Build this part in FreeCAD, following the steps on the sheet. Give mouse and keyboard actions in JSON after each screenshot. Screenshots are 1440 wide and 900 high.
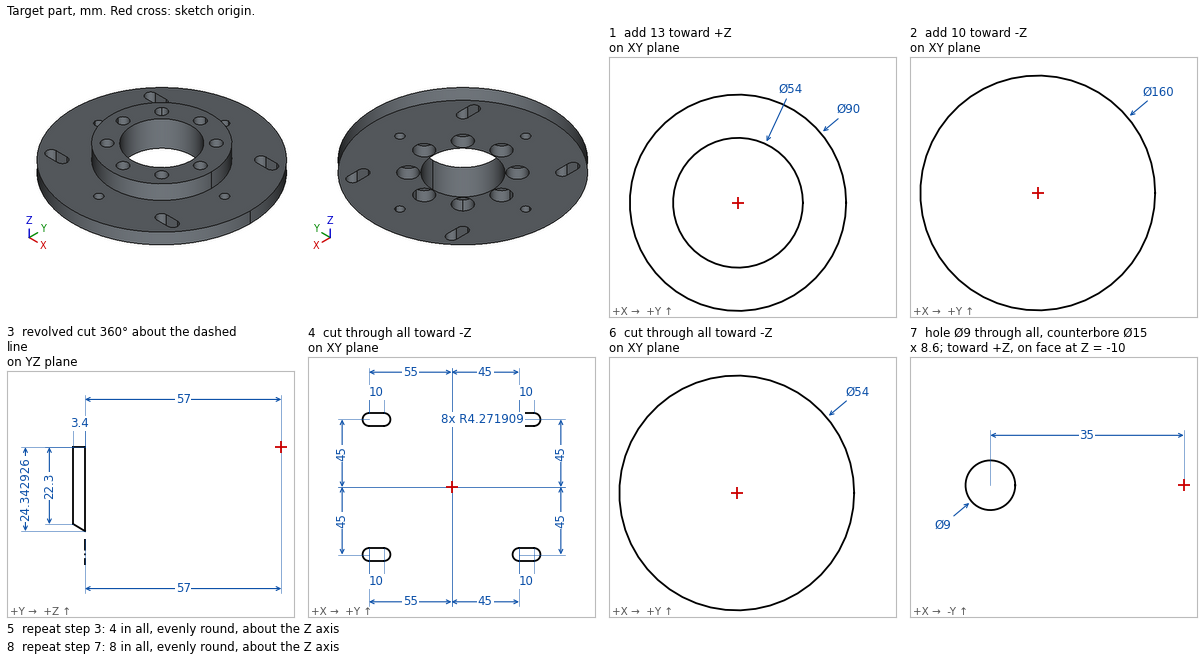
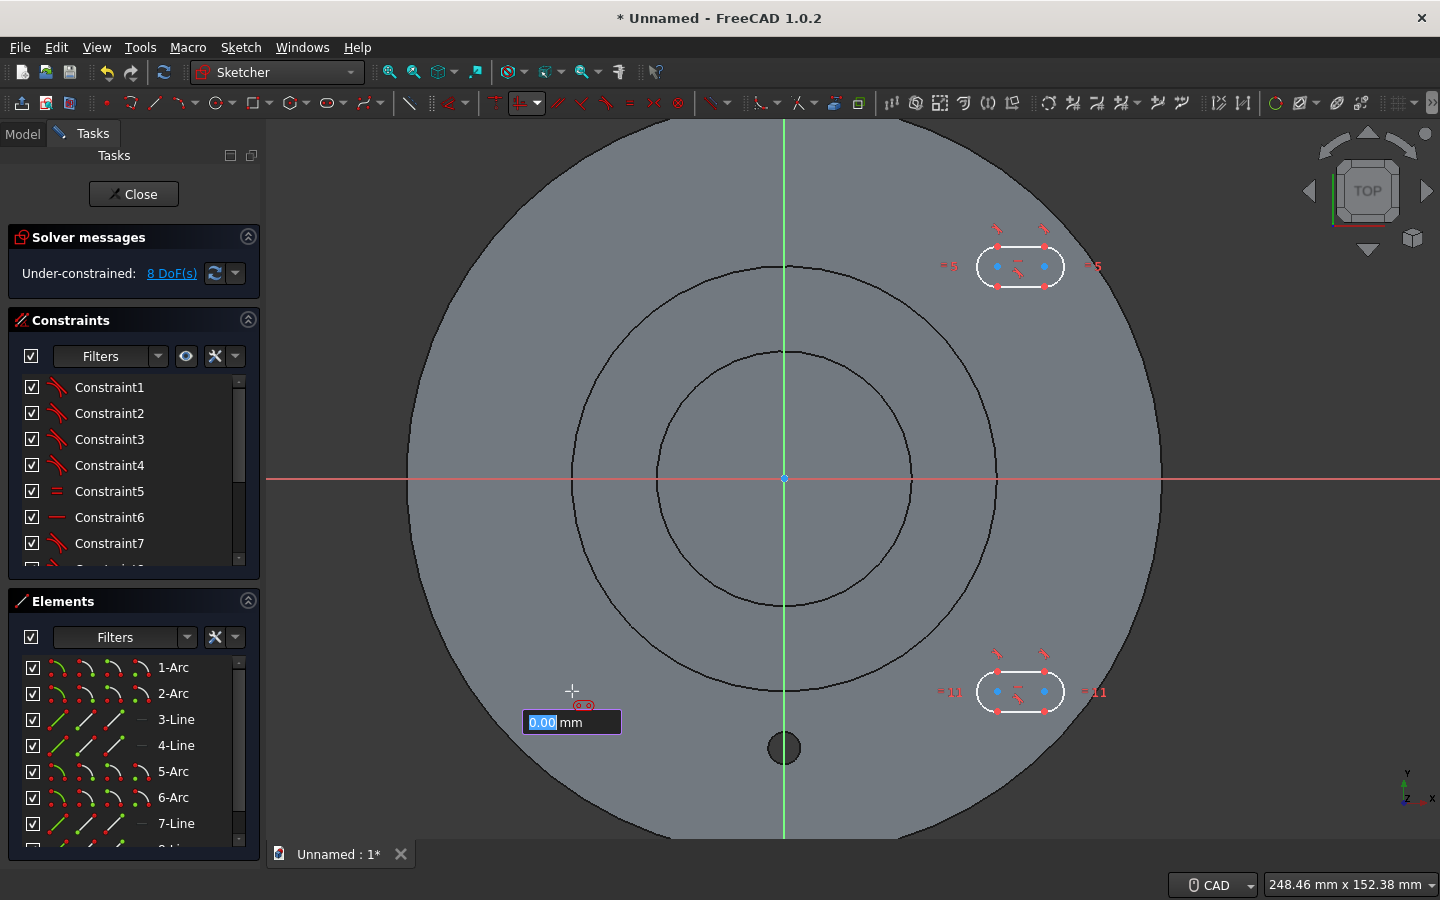
{"action": "left_click", "coordinate": [548, 671]}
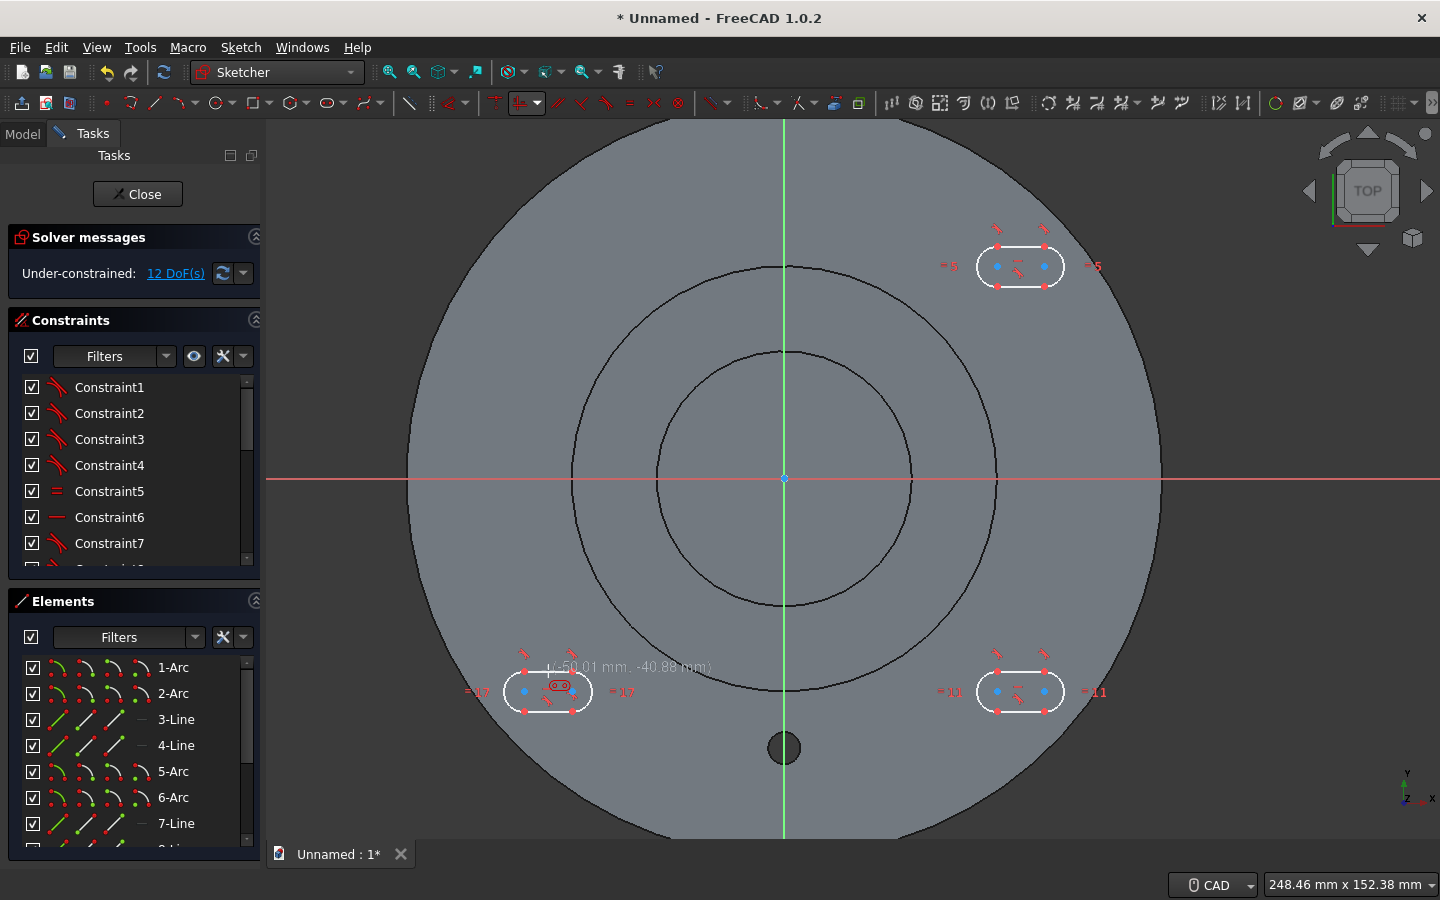
{"action": "left_click", "coordinate": [524, 266]}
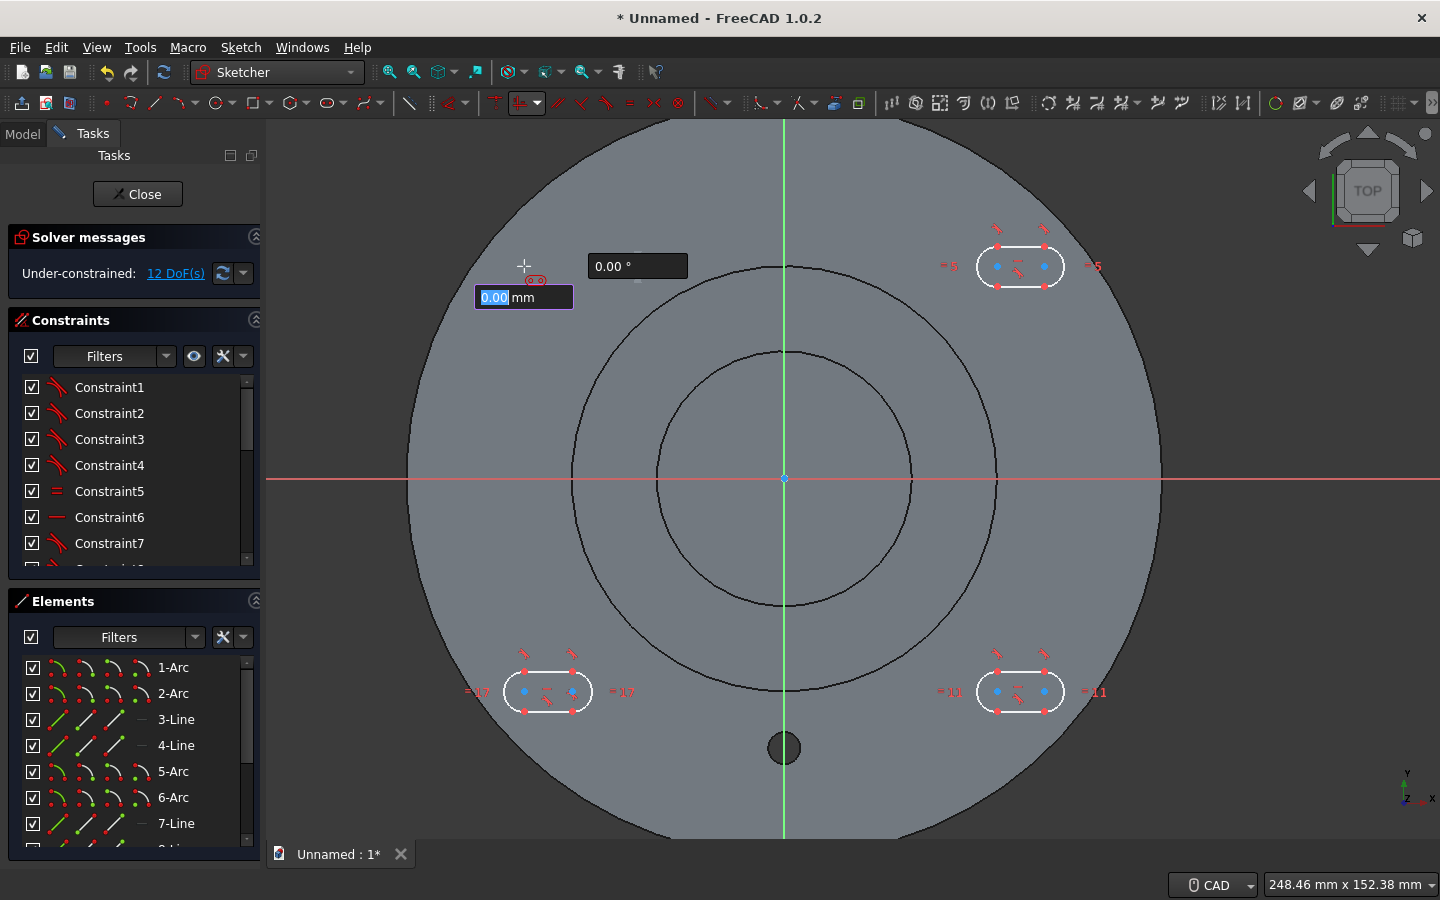
{"action": "left_click", "coordinate": [572, 266]}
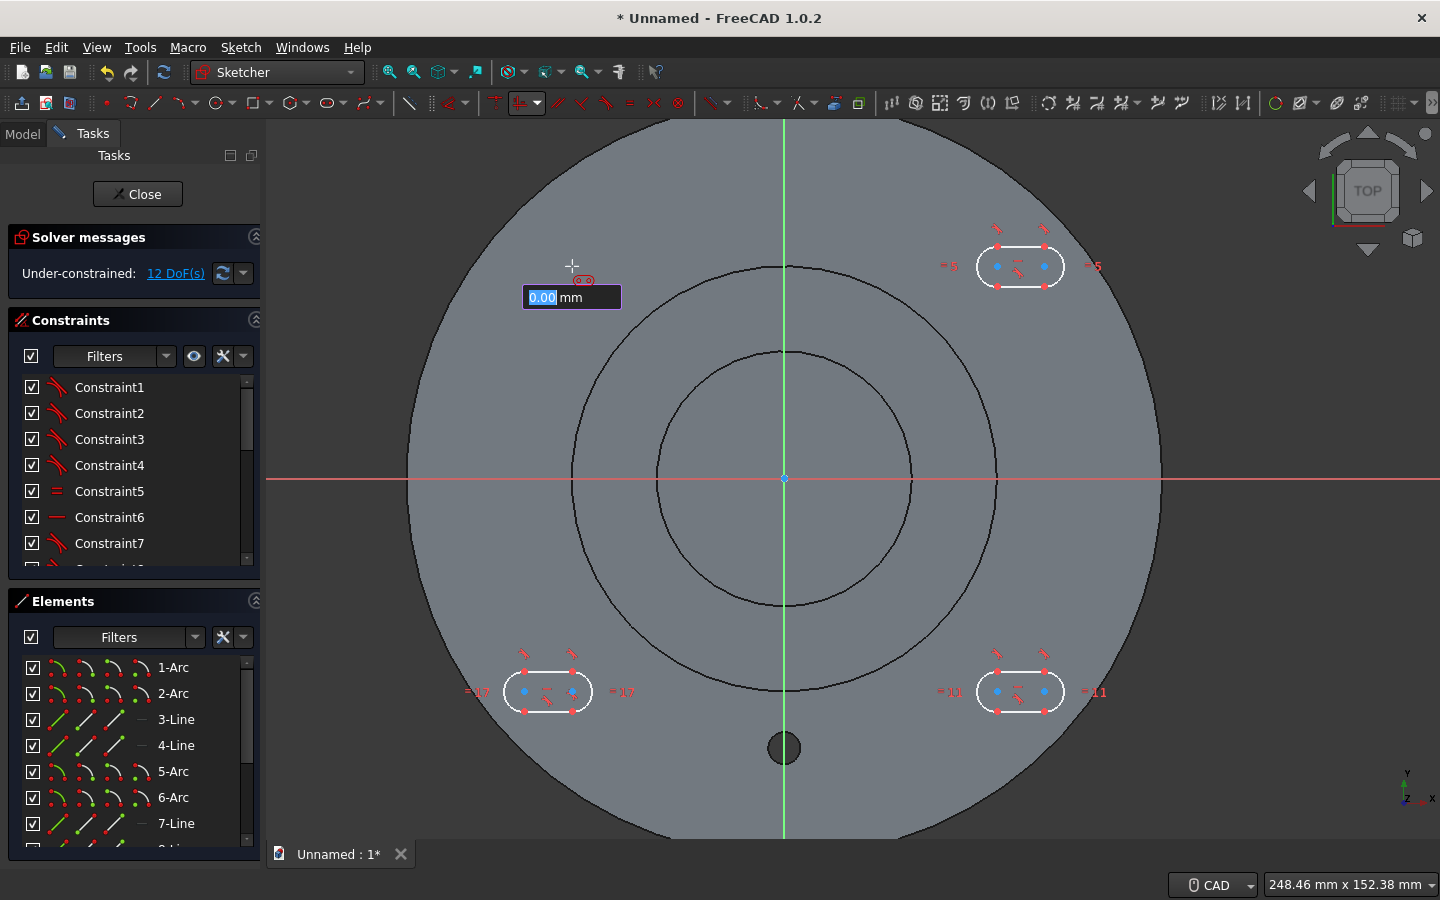
{"action": "left_click", "coordinate": [548, 246]}
{"action": "key", "text": "Escape"}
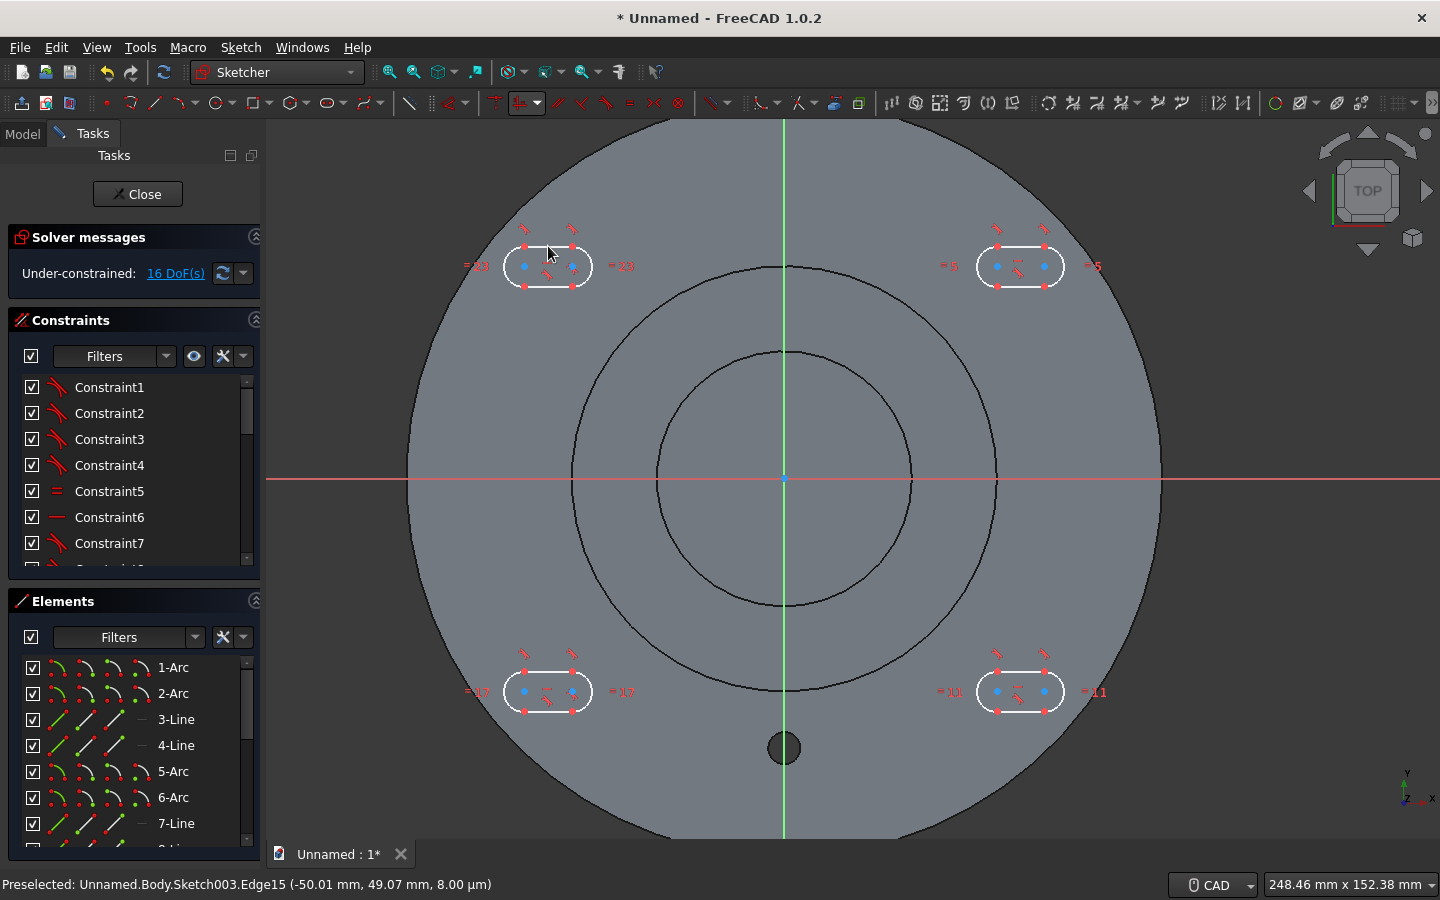
{"action": "left_click", "coordinate": [981, 255]}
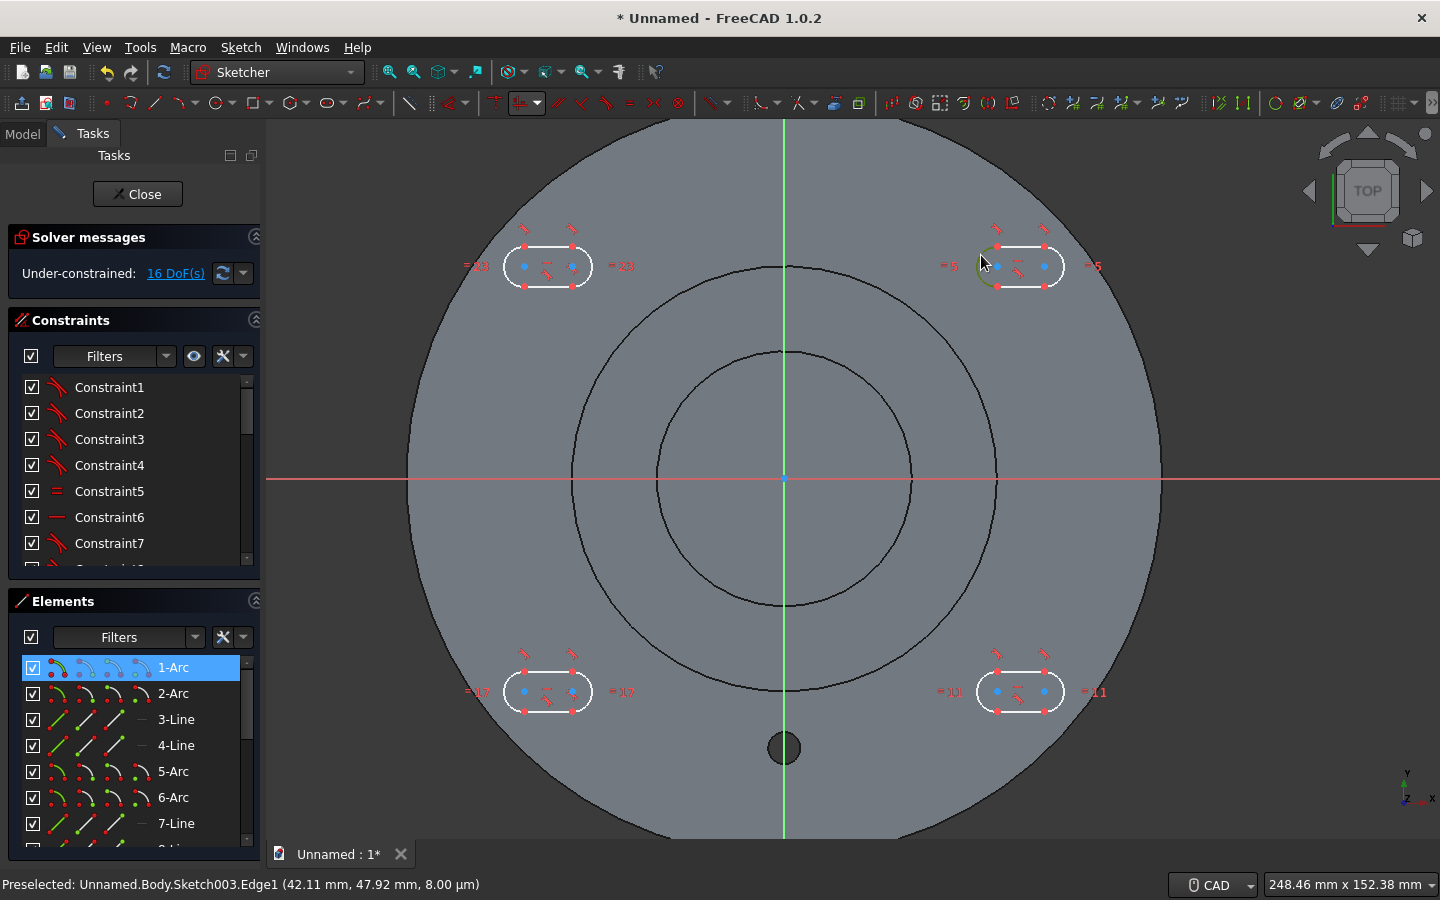
{"action": "left_click", "coordinate": [981, 680]}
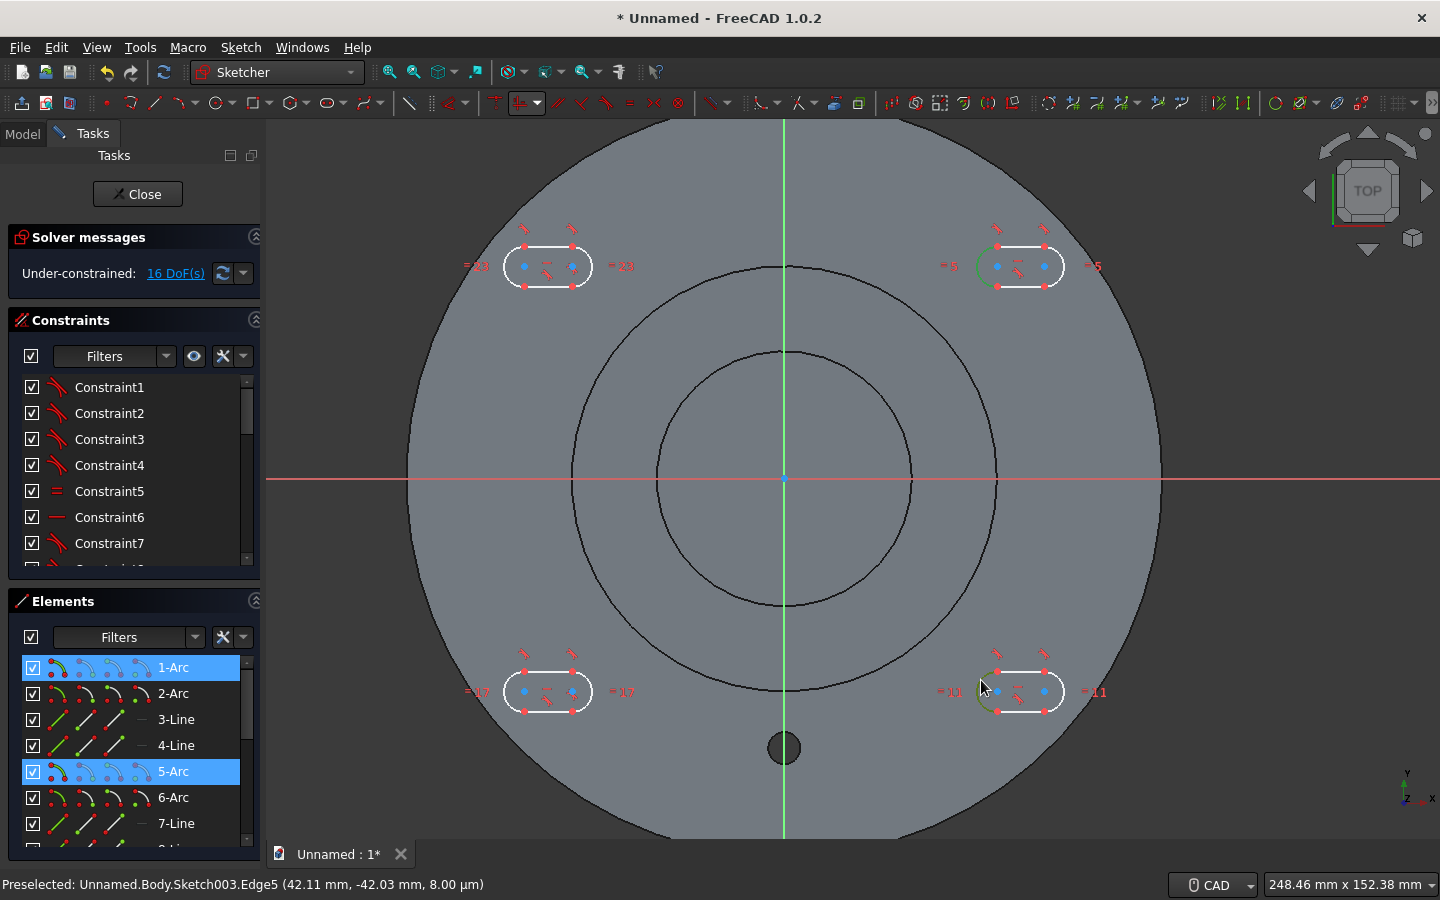
{"action": "left_click", "coordinate": [508, 680]}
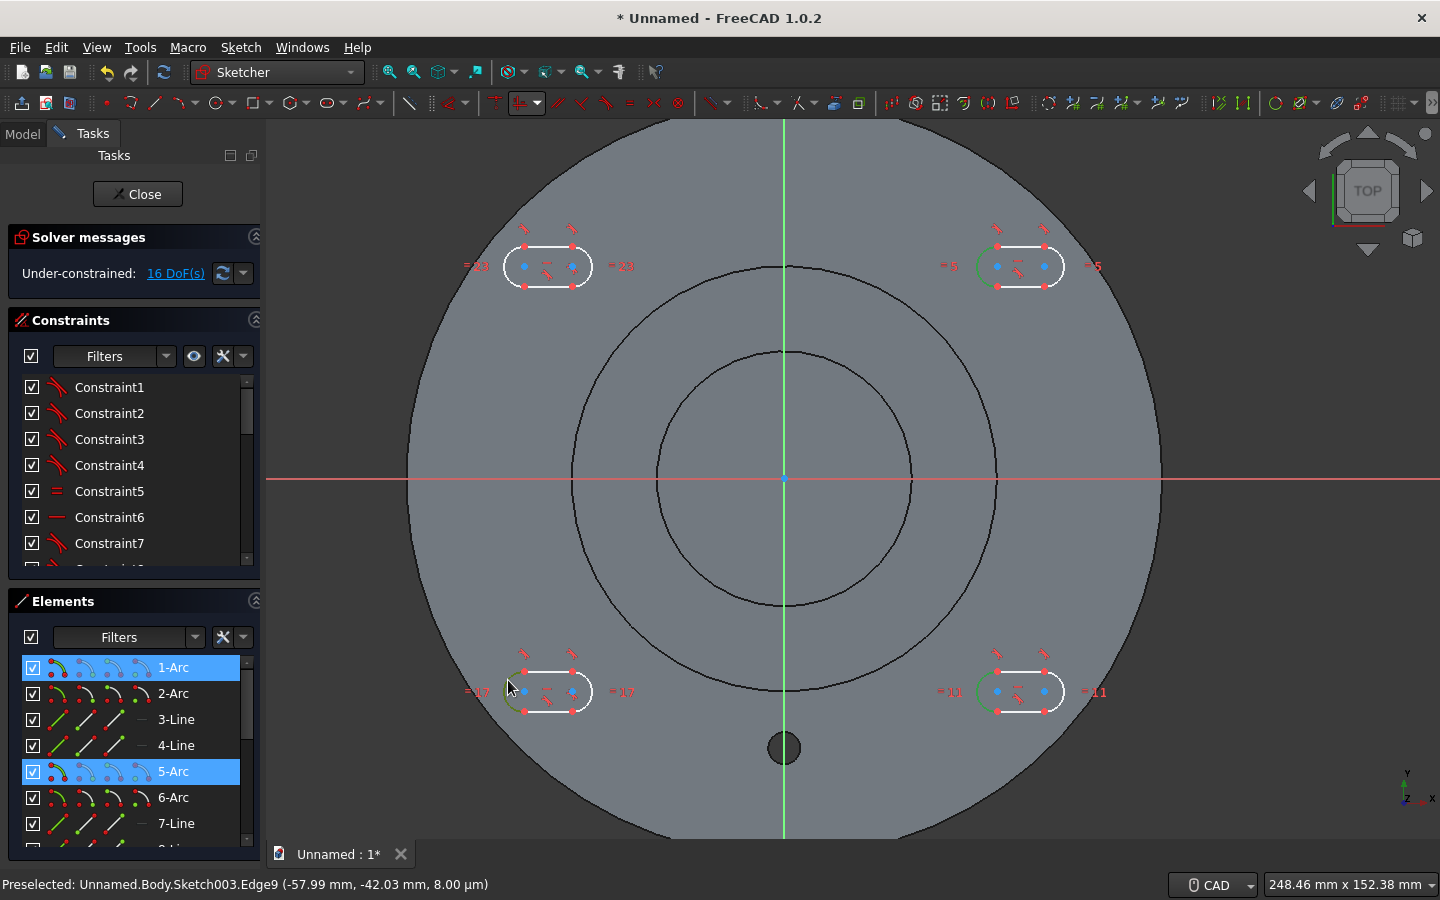
{"action": "left_click", "coordinate": [508, 255]}